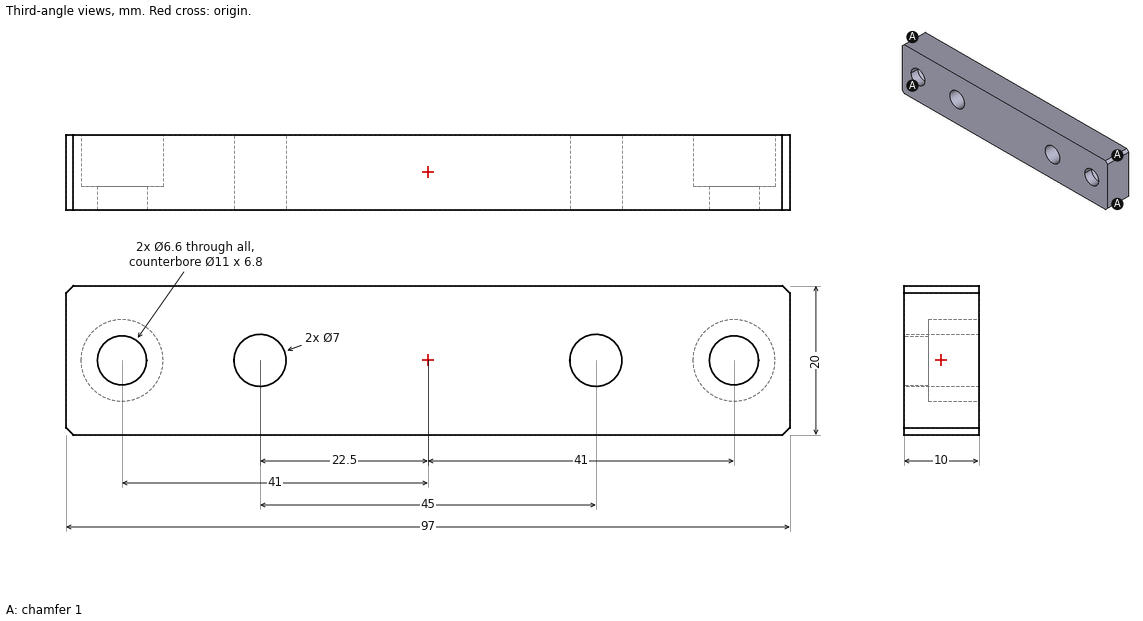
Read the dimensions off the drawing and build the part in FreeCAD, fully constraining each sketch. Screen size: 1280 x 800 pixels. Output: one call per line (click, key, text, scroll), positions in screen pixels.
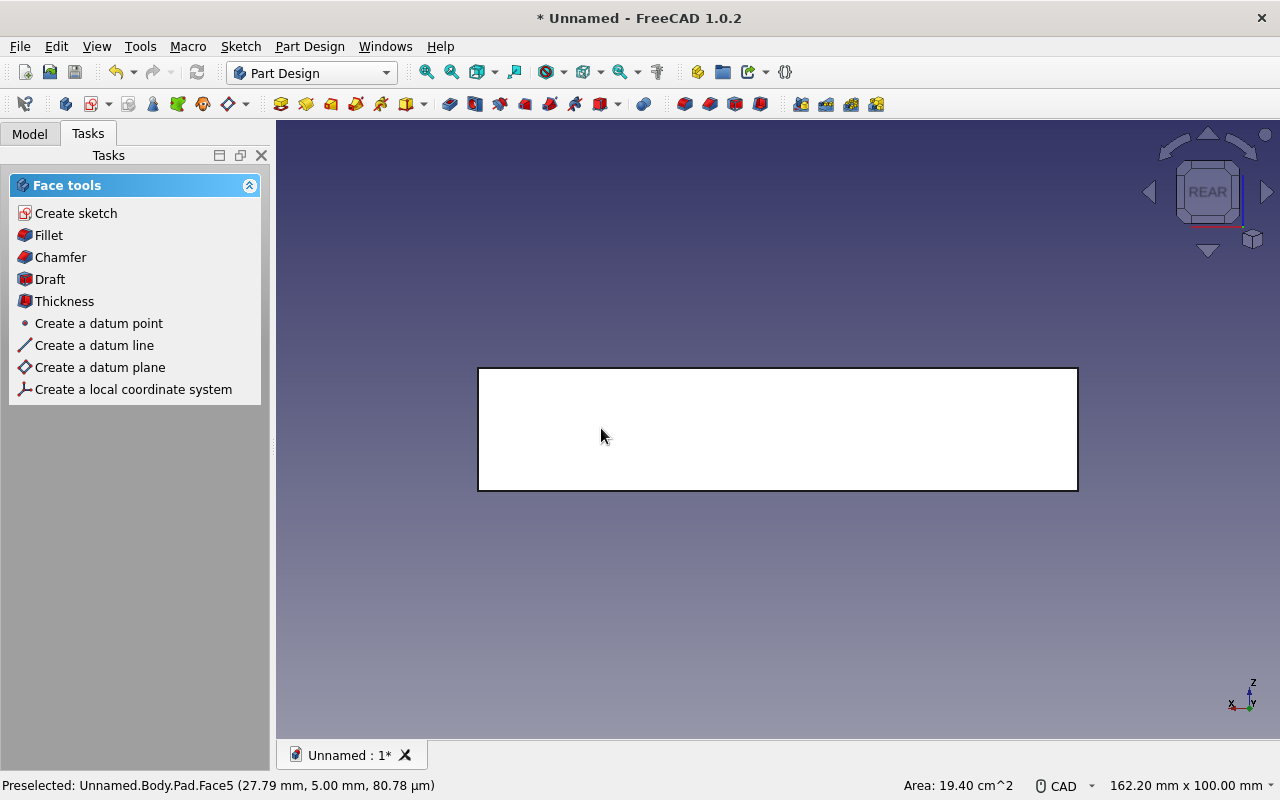
click(90, 104)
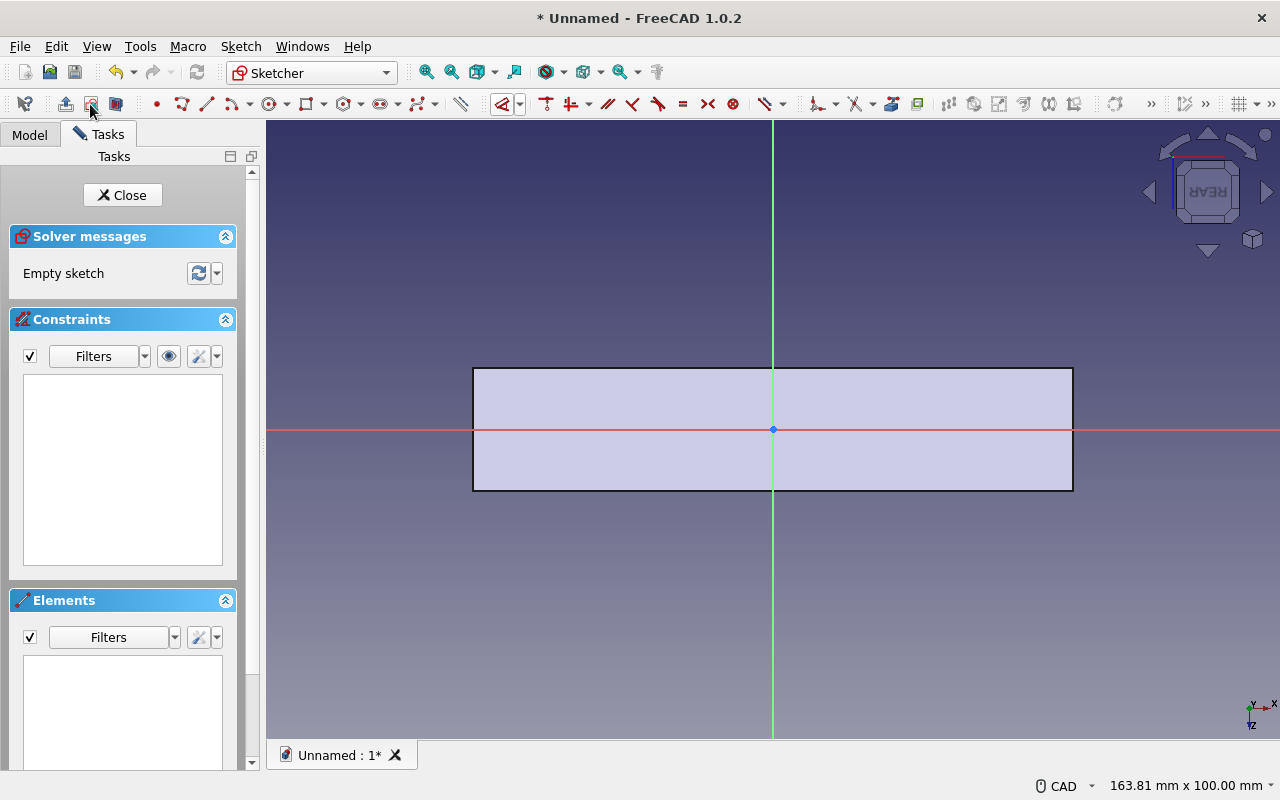
scroll(856, 430, up, 3)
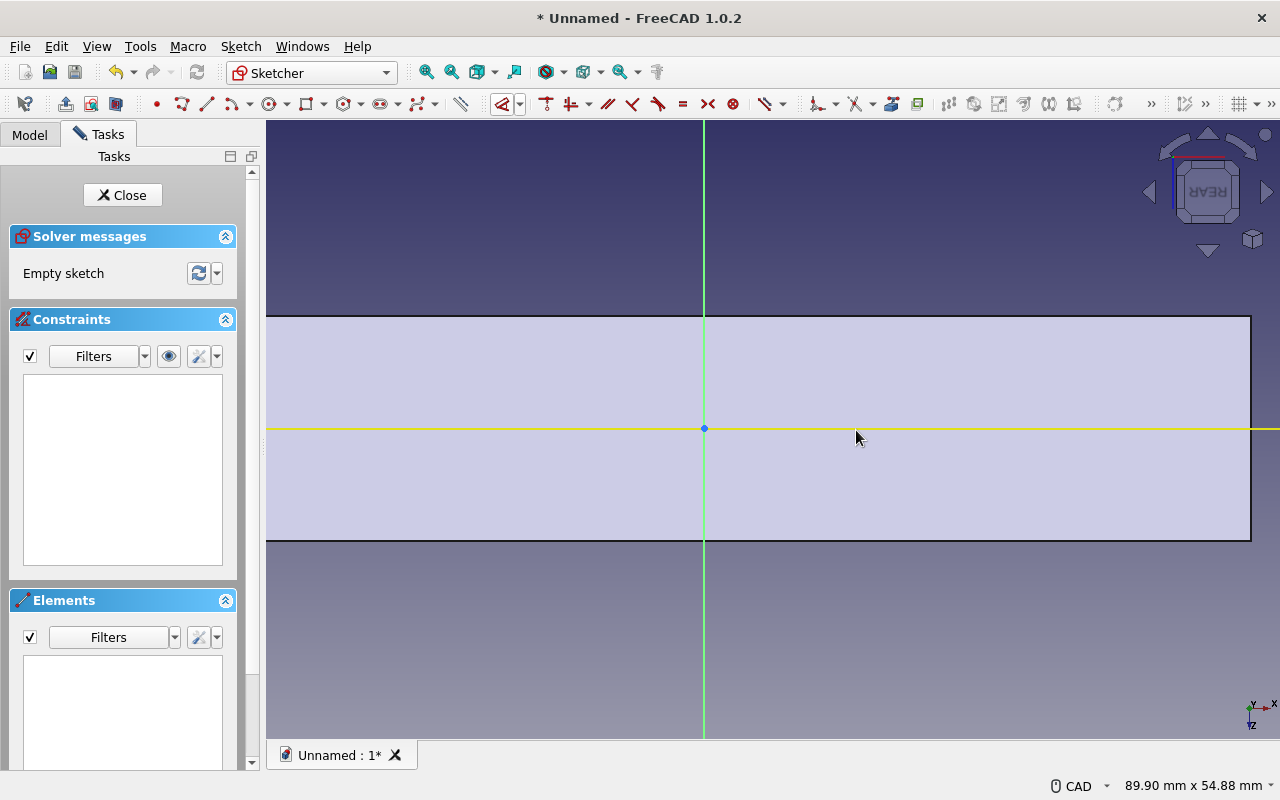
click(268, 104)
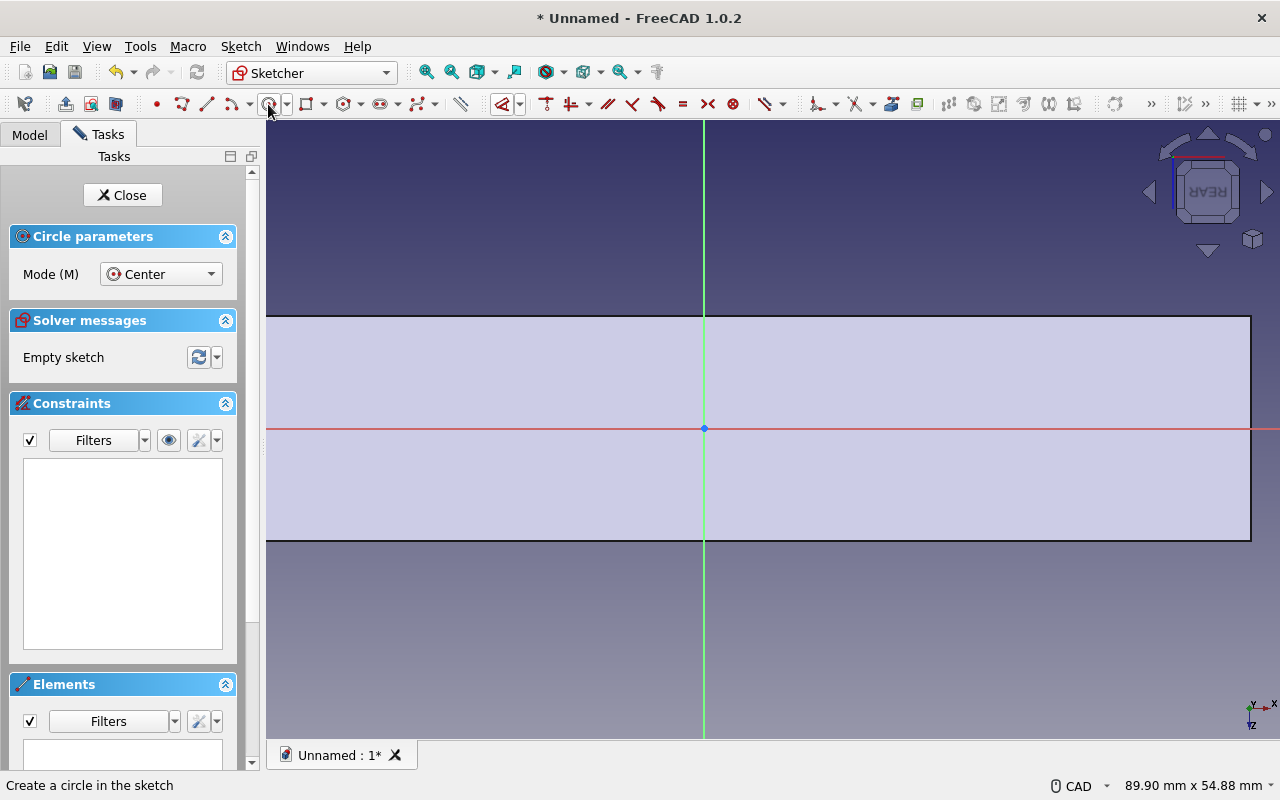
click(451, 429)
click(478, 401)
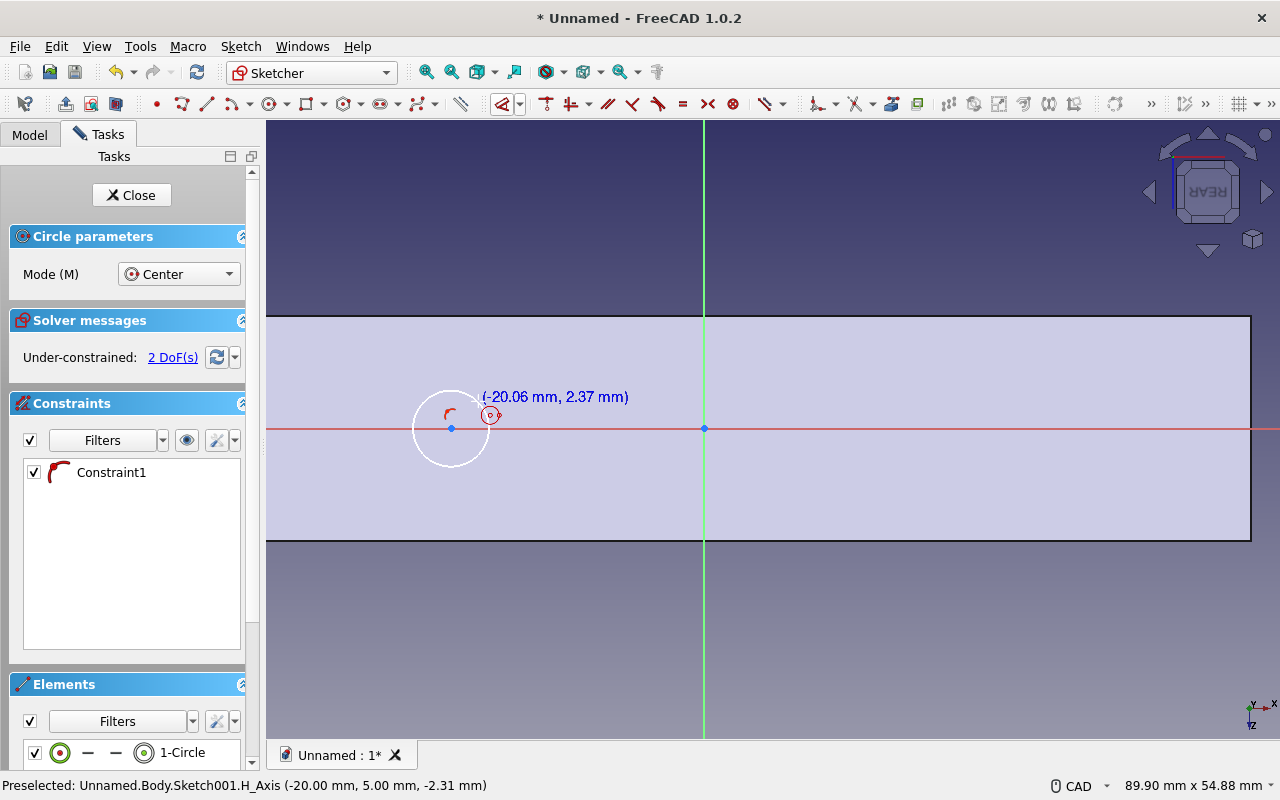
click(958, 429)
click(986, 401)
key(Escape)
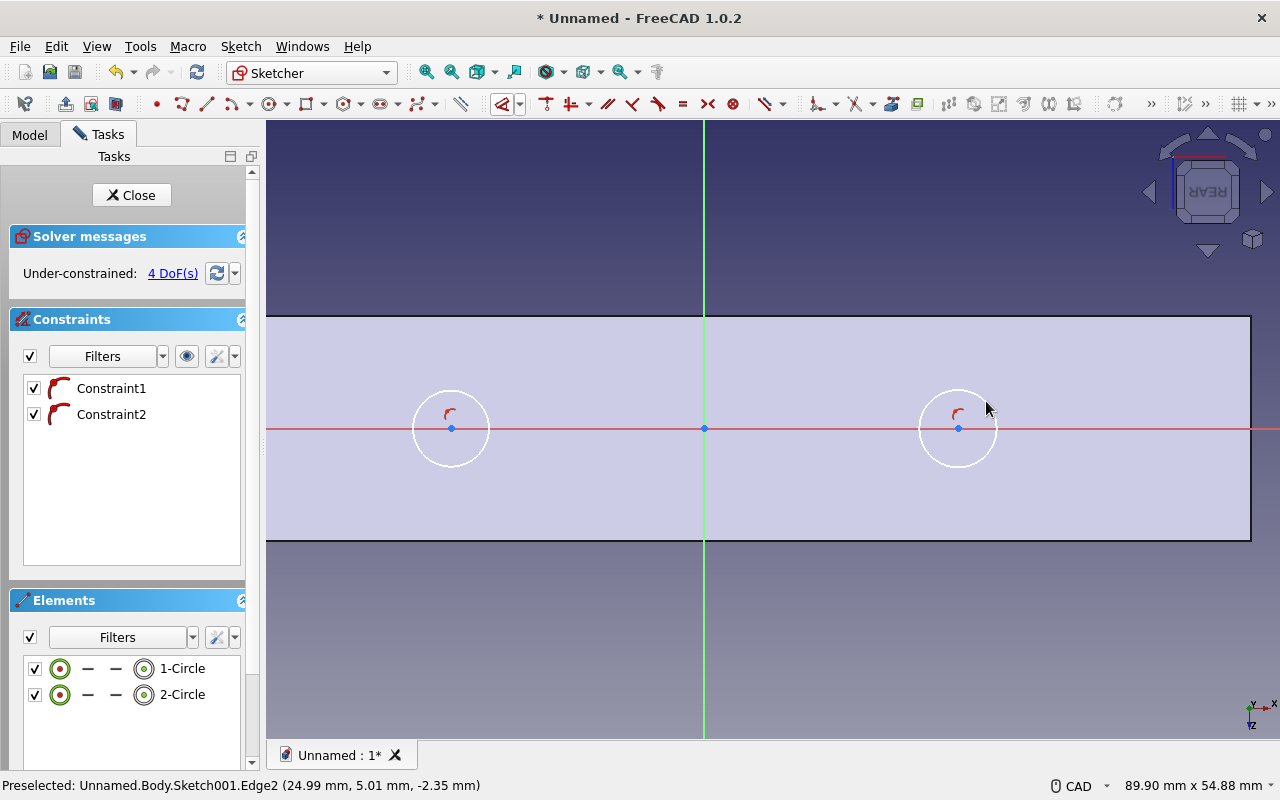
click(478, 402)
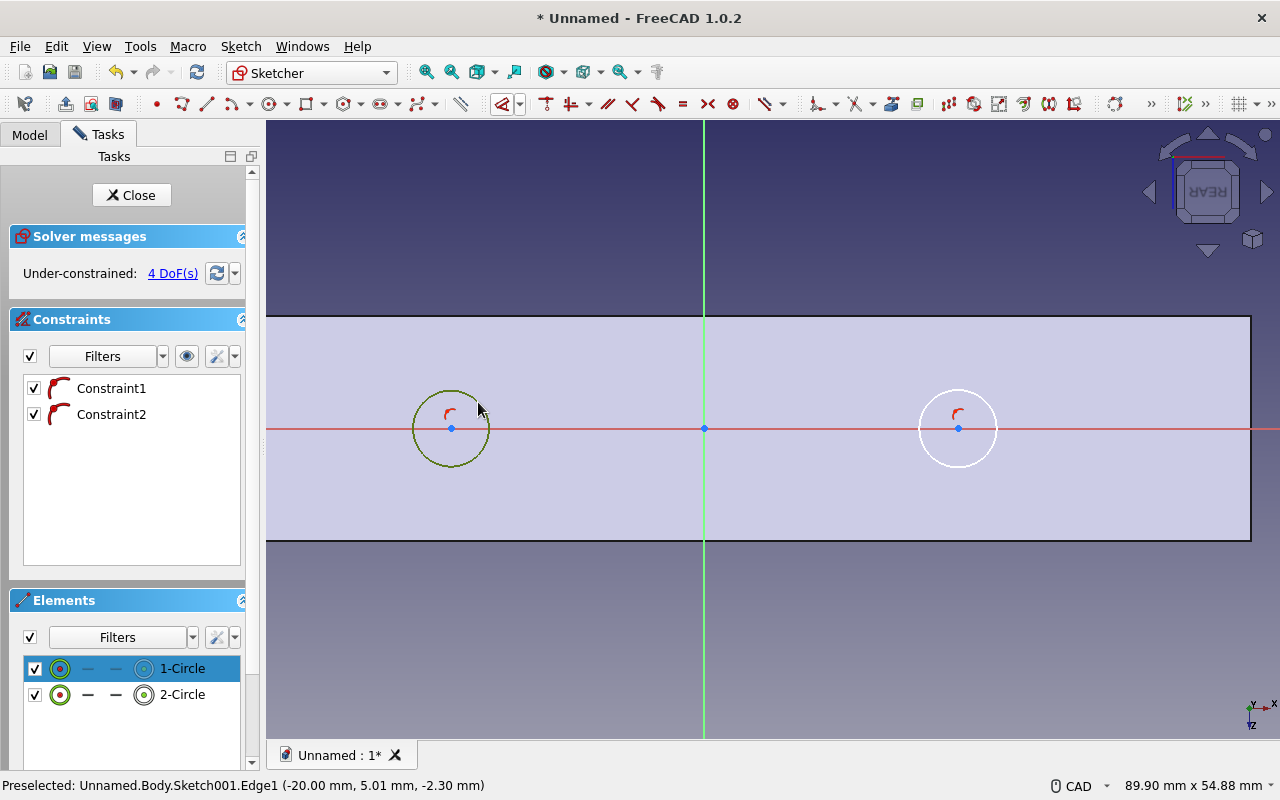
click(985, 401)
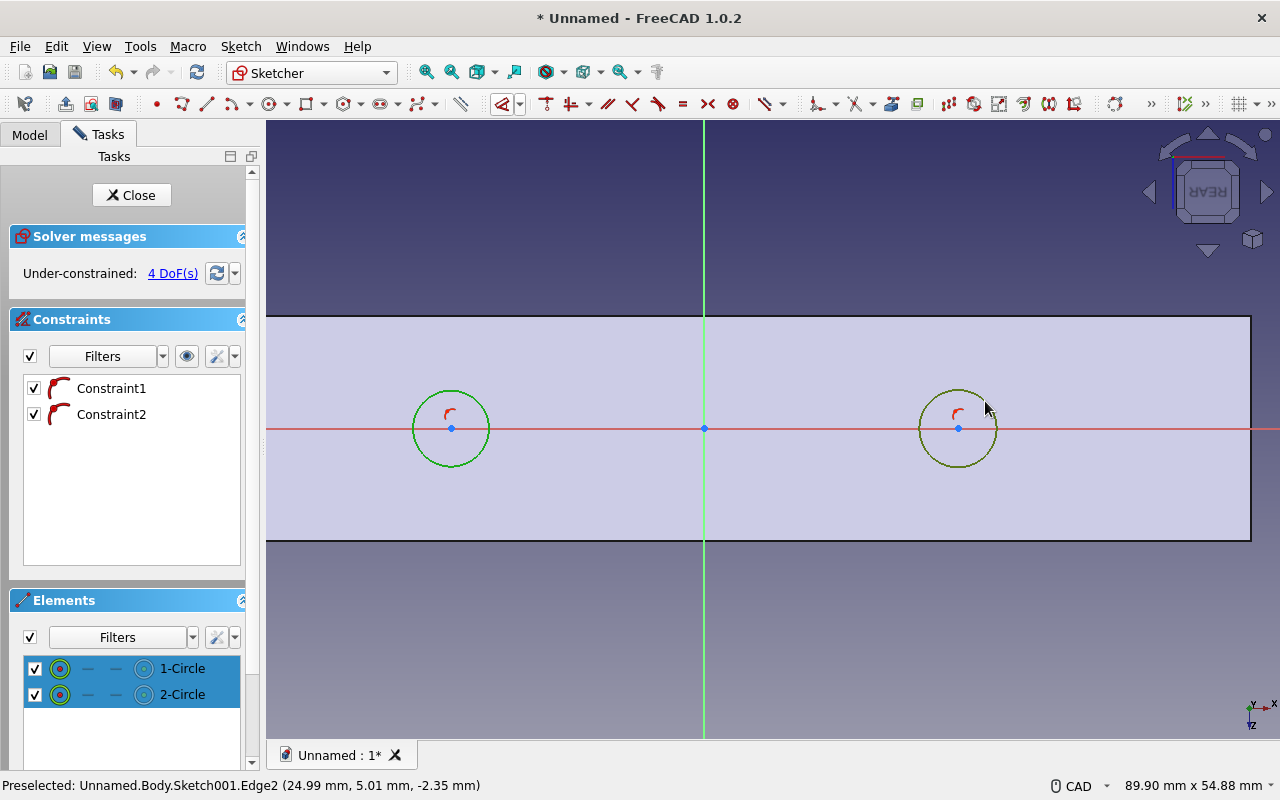
click(683, 104)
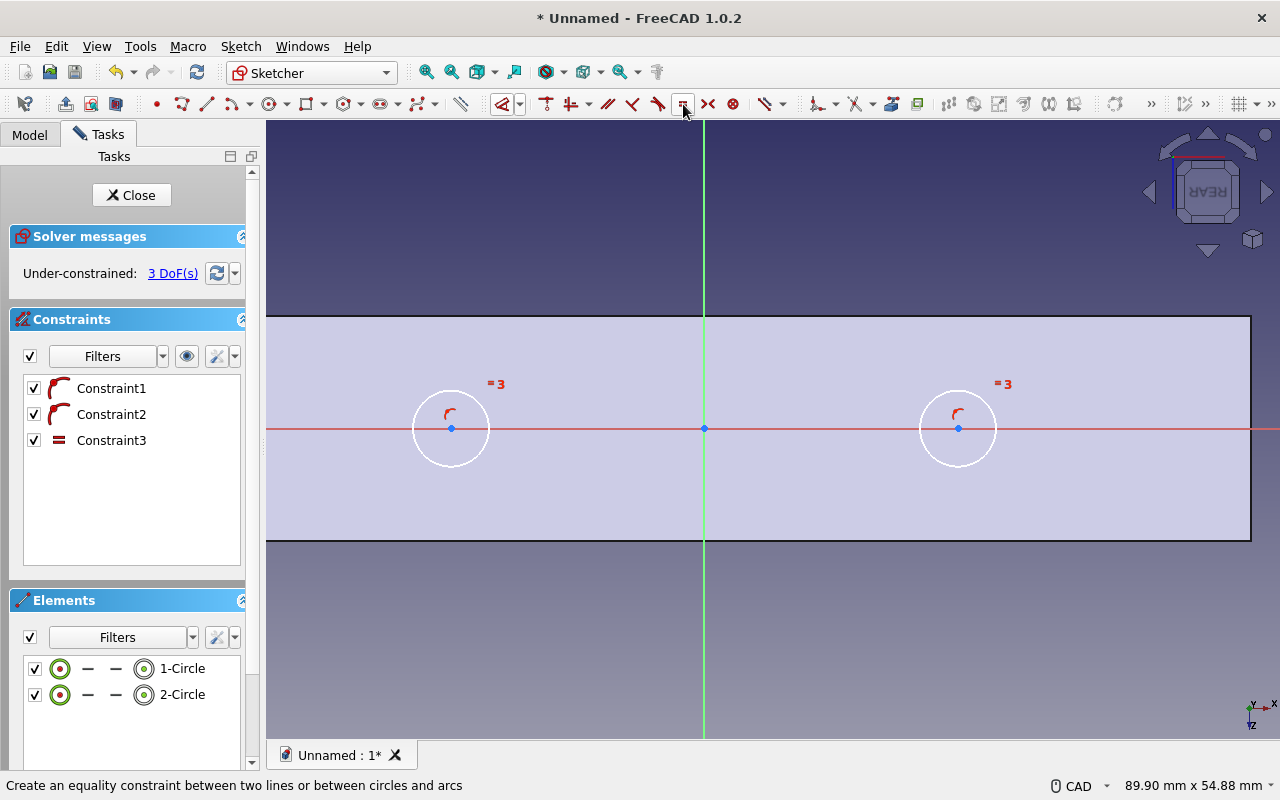
click(478, 402)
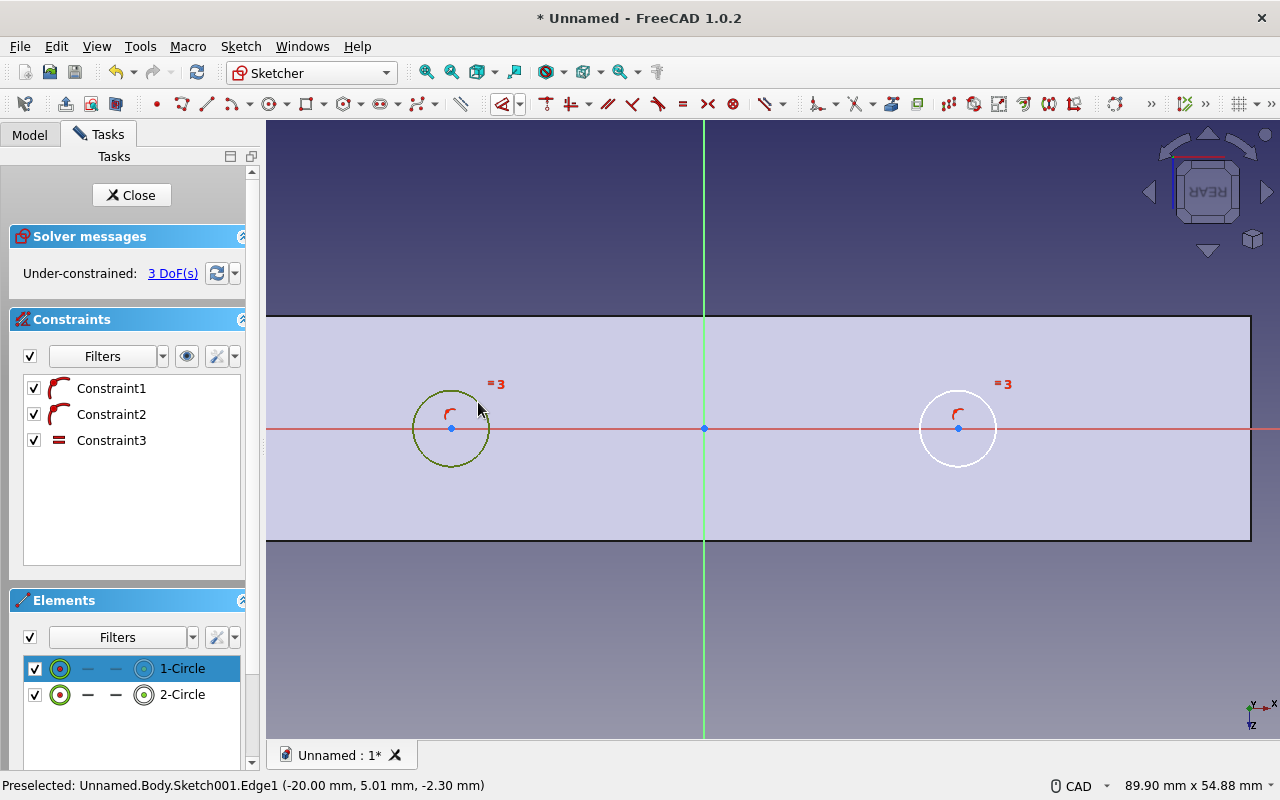
key(k)
key(o)